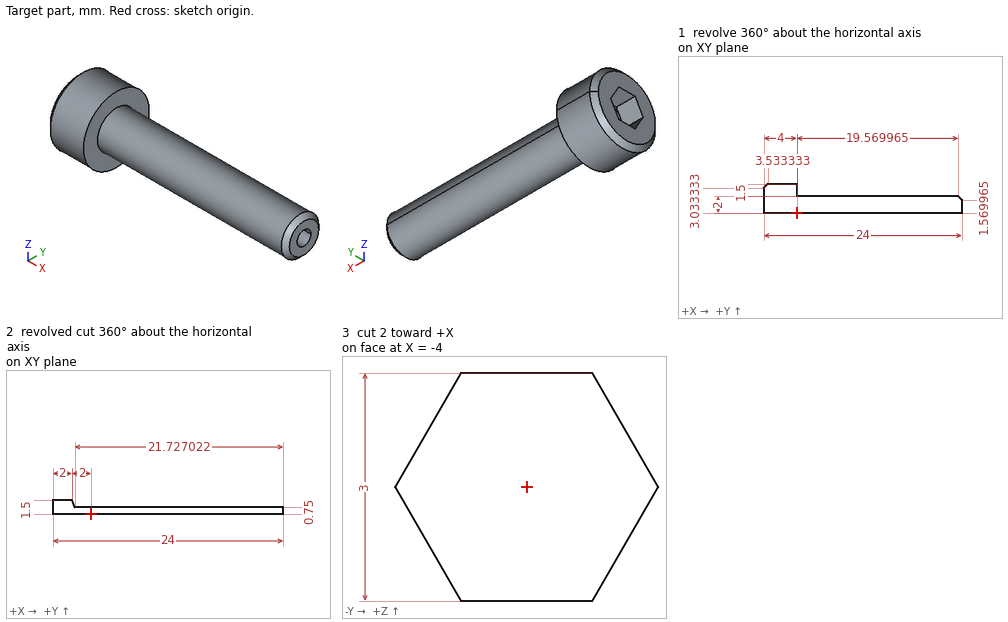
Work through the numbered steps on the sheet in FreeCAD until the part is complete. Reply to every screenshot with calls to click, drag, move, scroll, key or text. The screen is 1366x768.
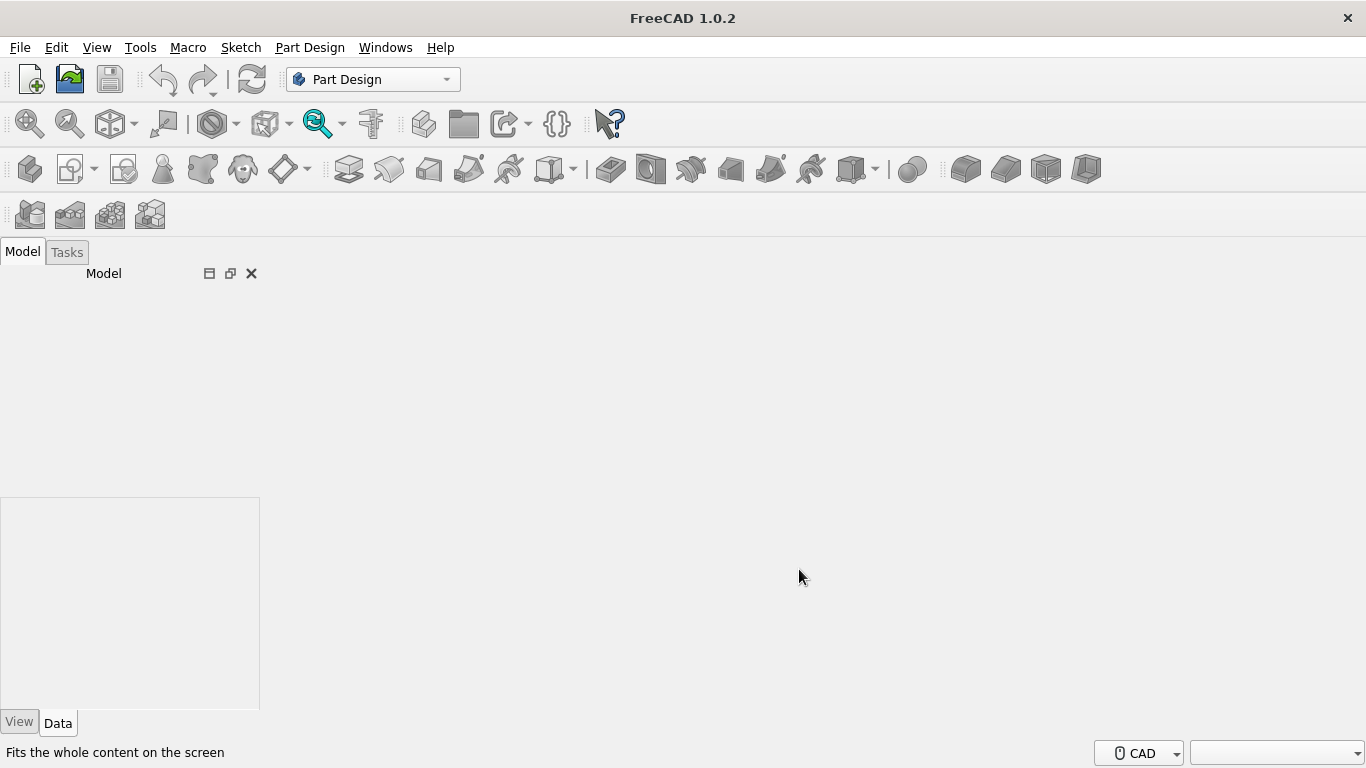
click(30, 80)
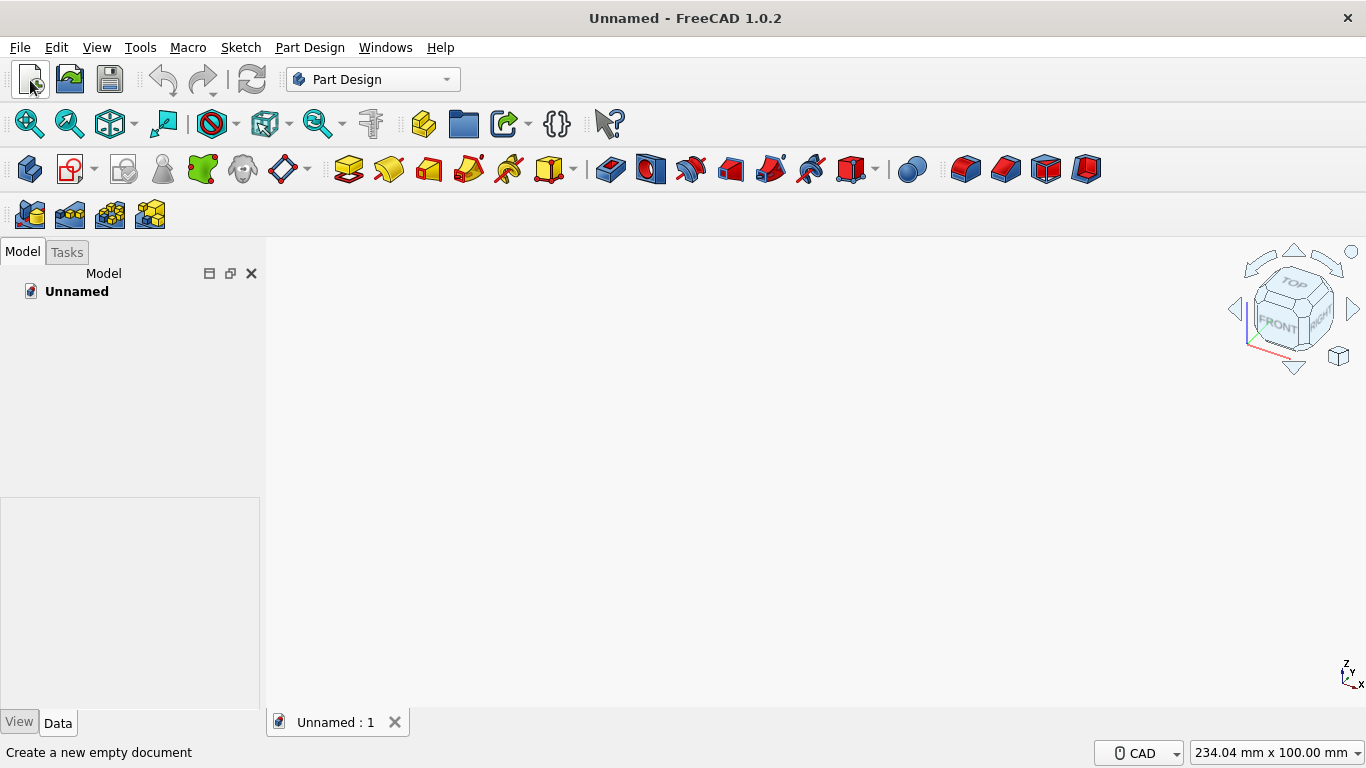
click(70, 170)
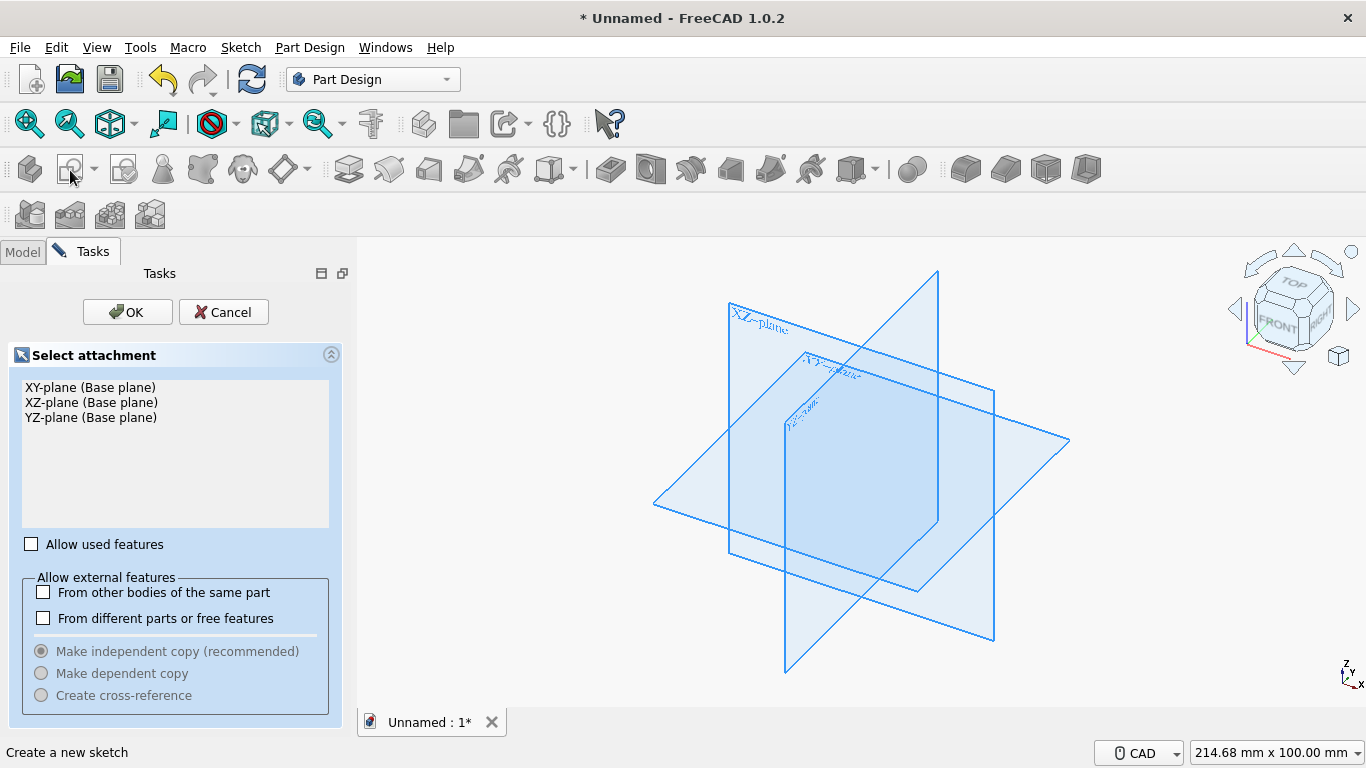
click(82, 388)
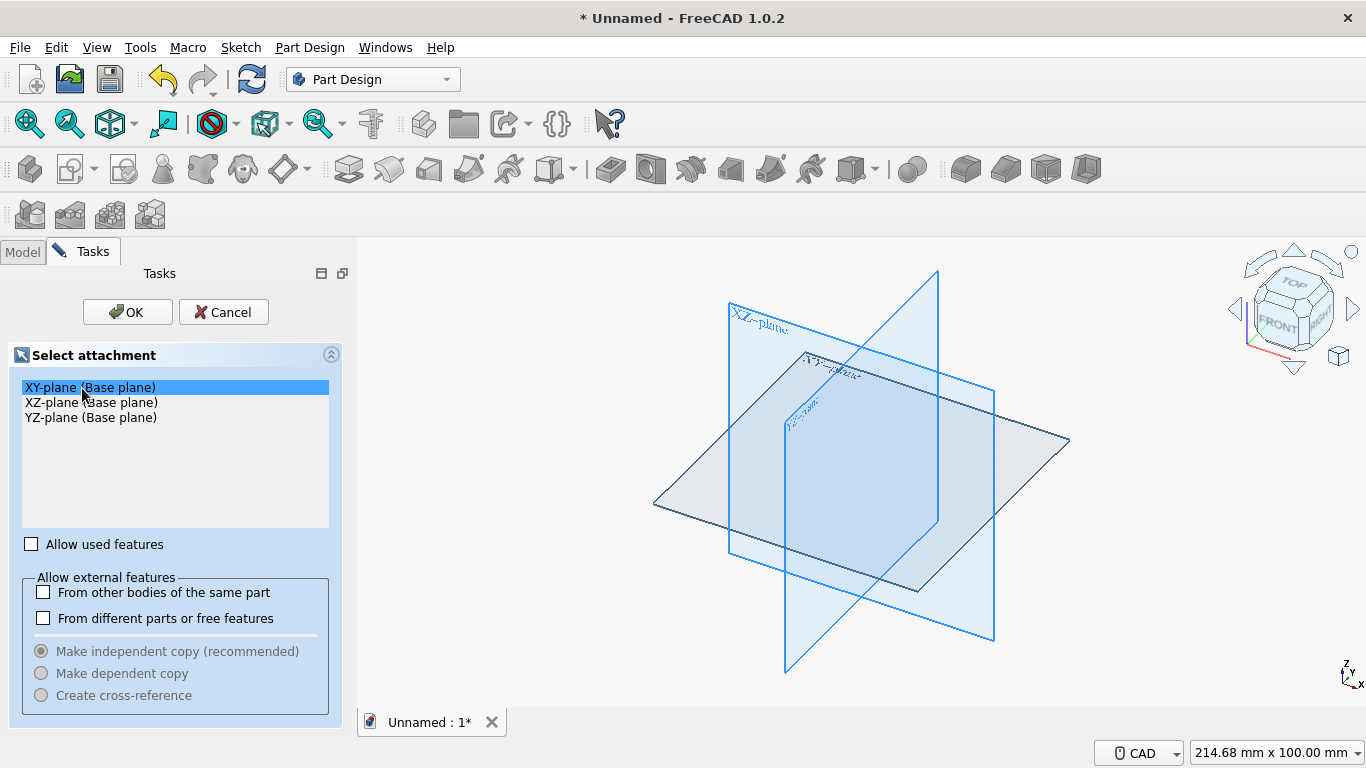
click(128, 312)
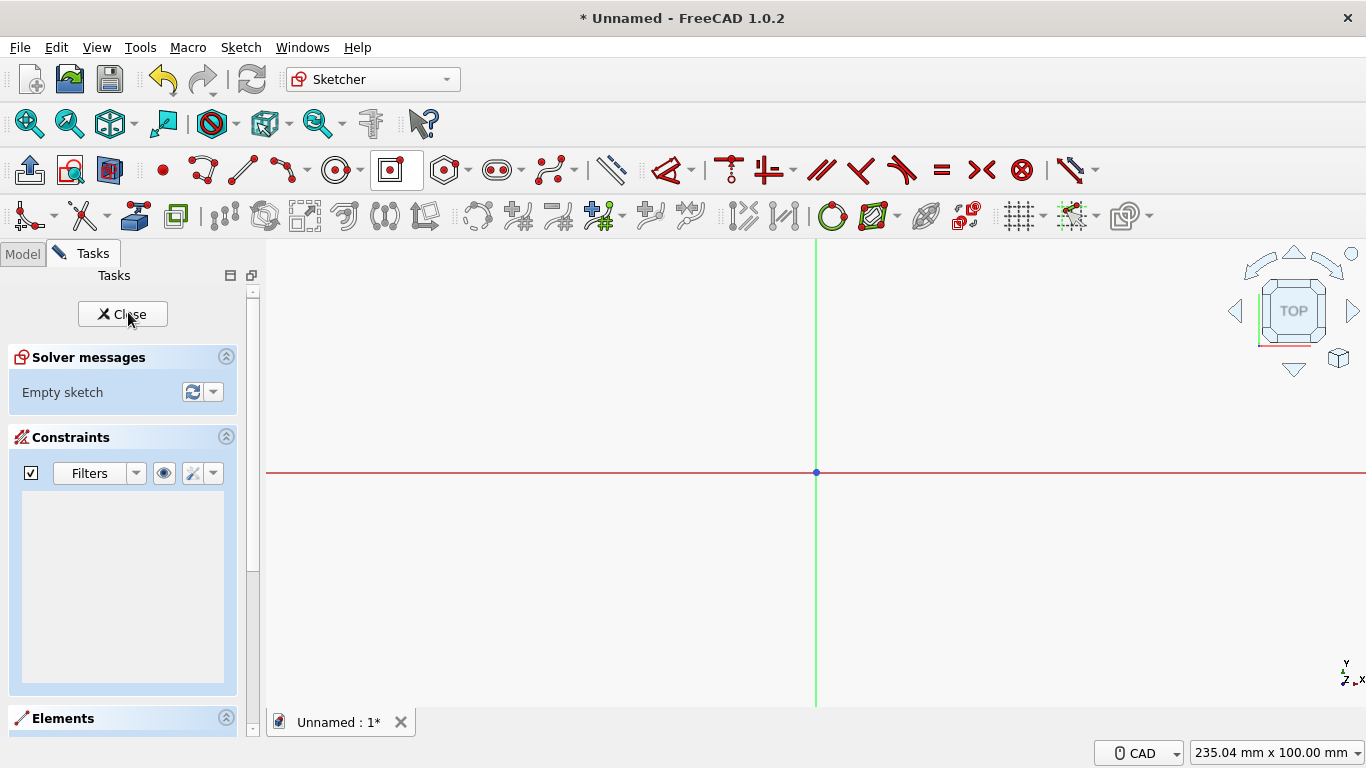
scroll(874, 463, up, 9)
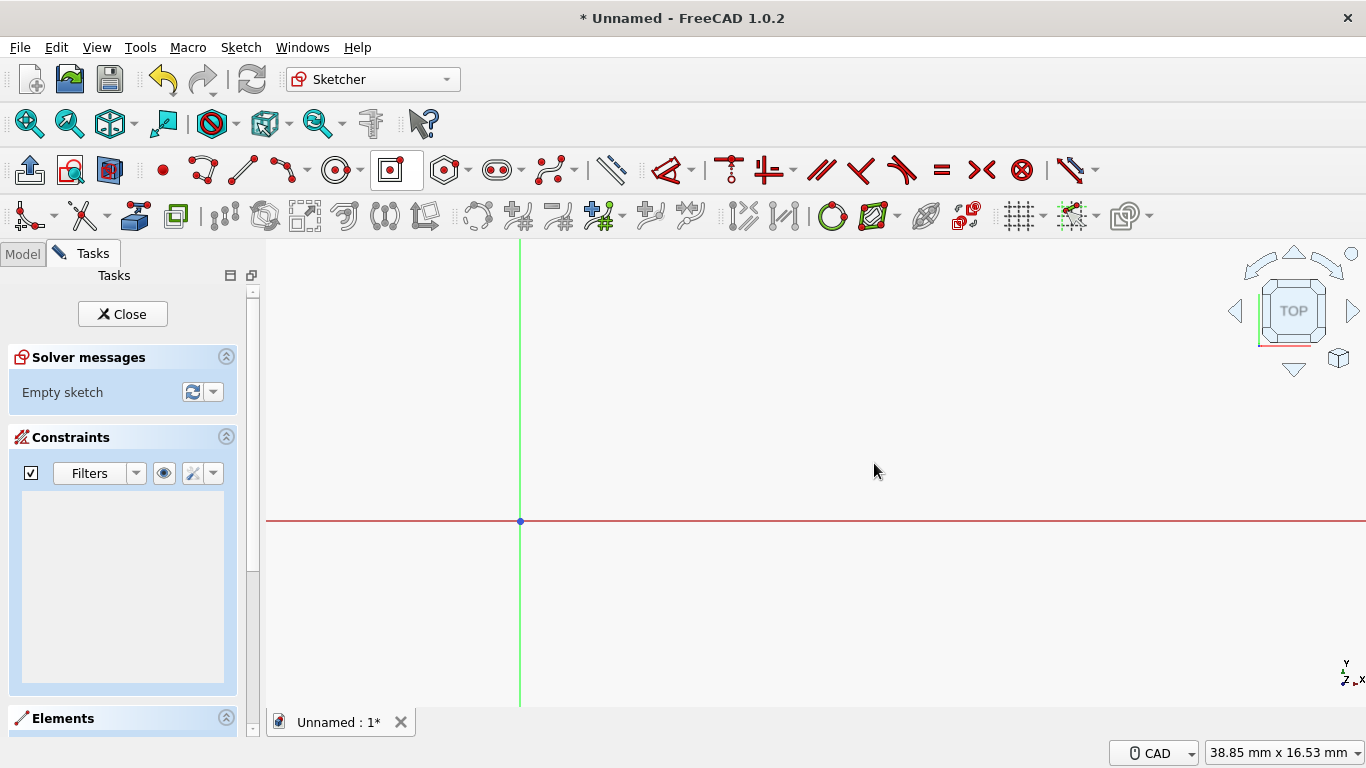
click(204, 170)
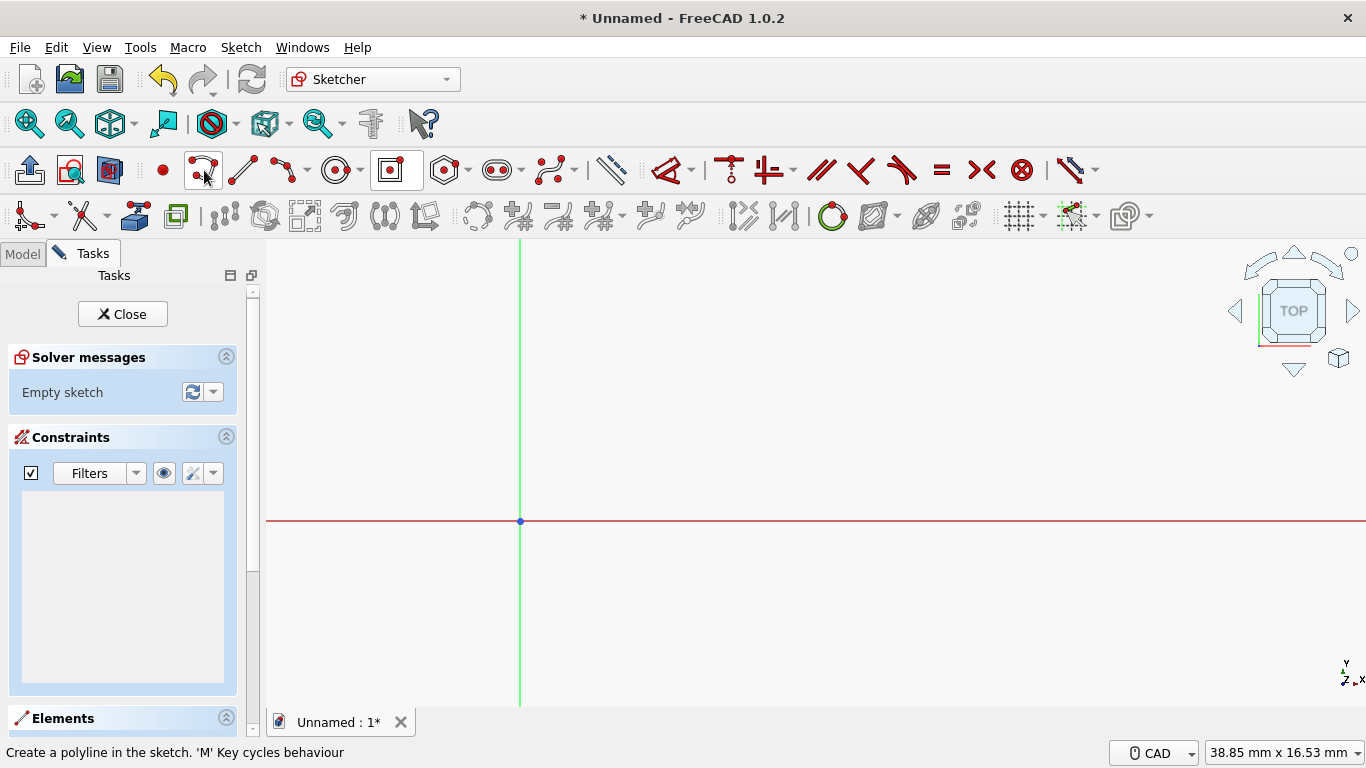
click(520, 464)
click(529, 422)
click(420, 422)
click(407, 435)
click(407, 521)
click(1087, 512)
click(1087, 477)
click(1074, 464)
click(520, 465)
key(Escape)
key(Escape)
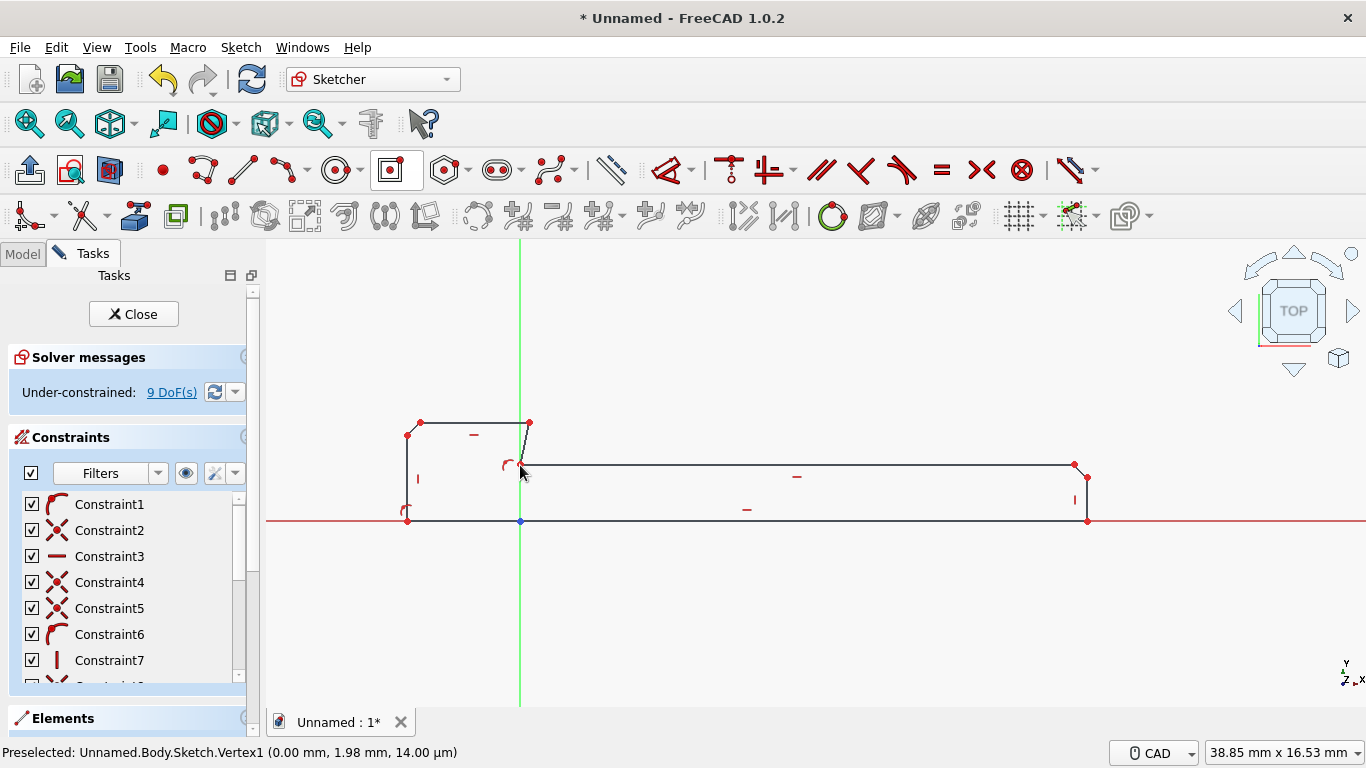
click(523, 452)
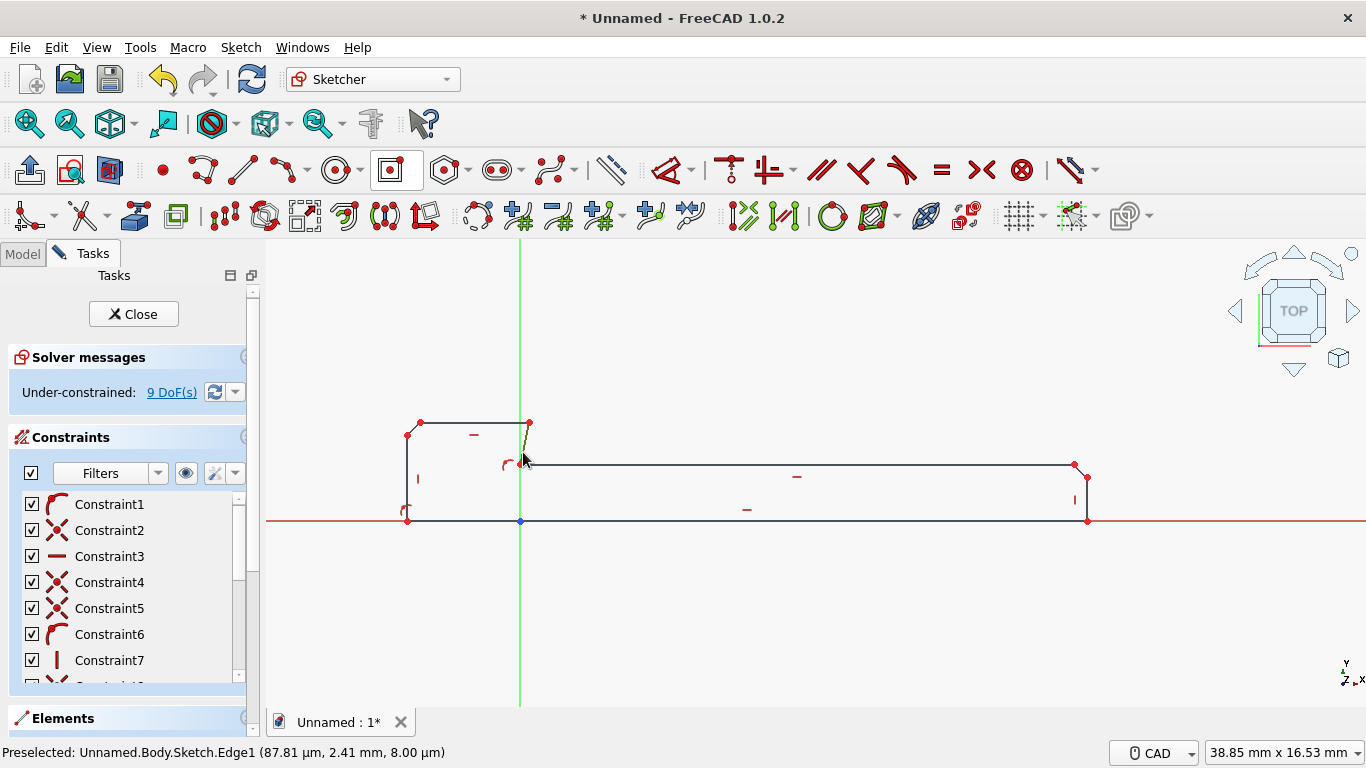
click(796, 170)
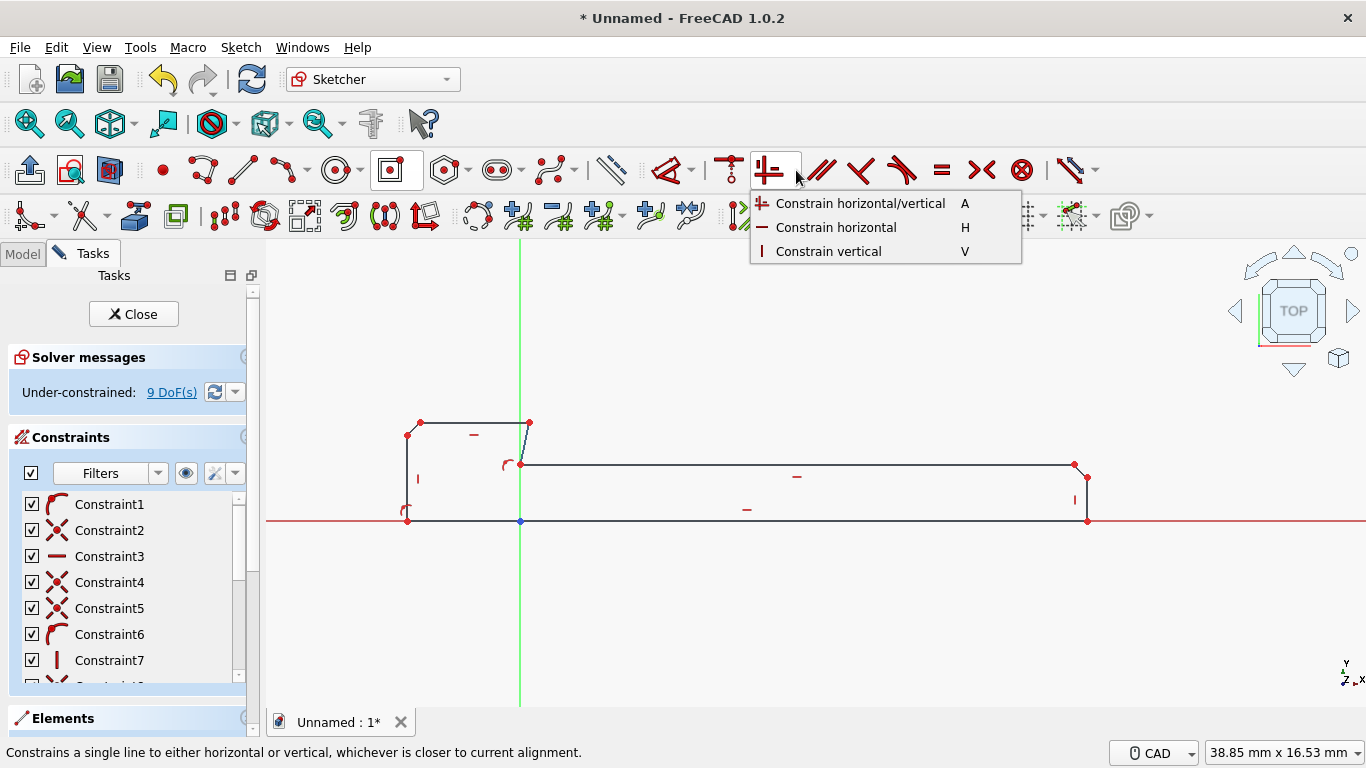
click(886, 251)